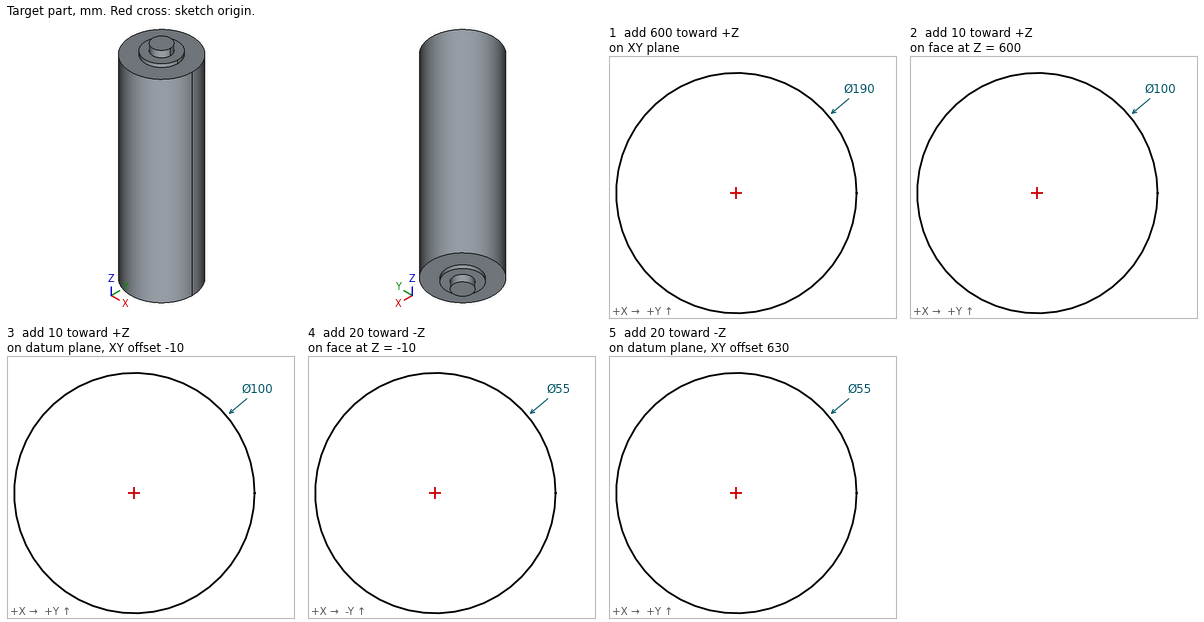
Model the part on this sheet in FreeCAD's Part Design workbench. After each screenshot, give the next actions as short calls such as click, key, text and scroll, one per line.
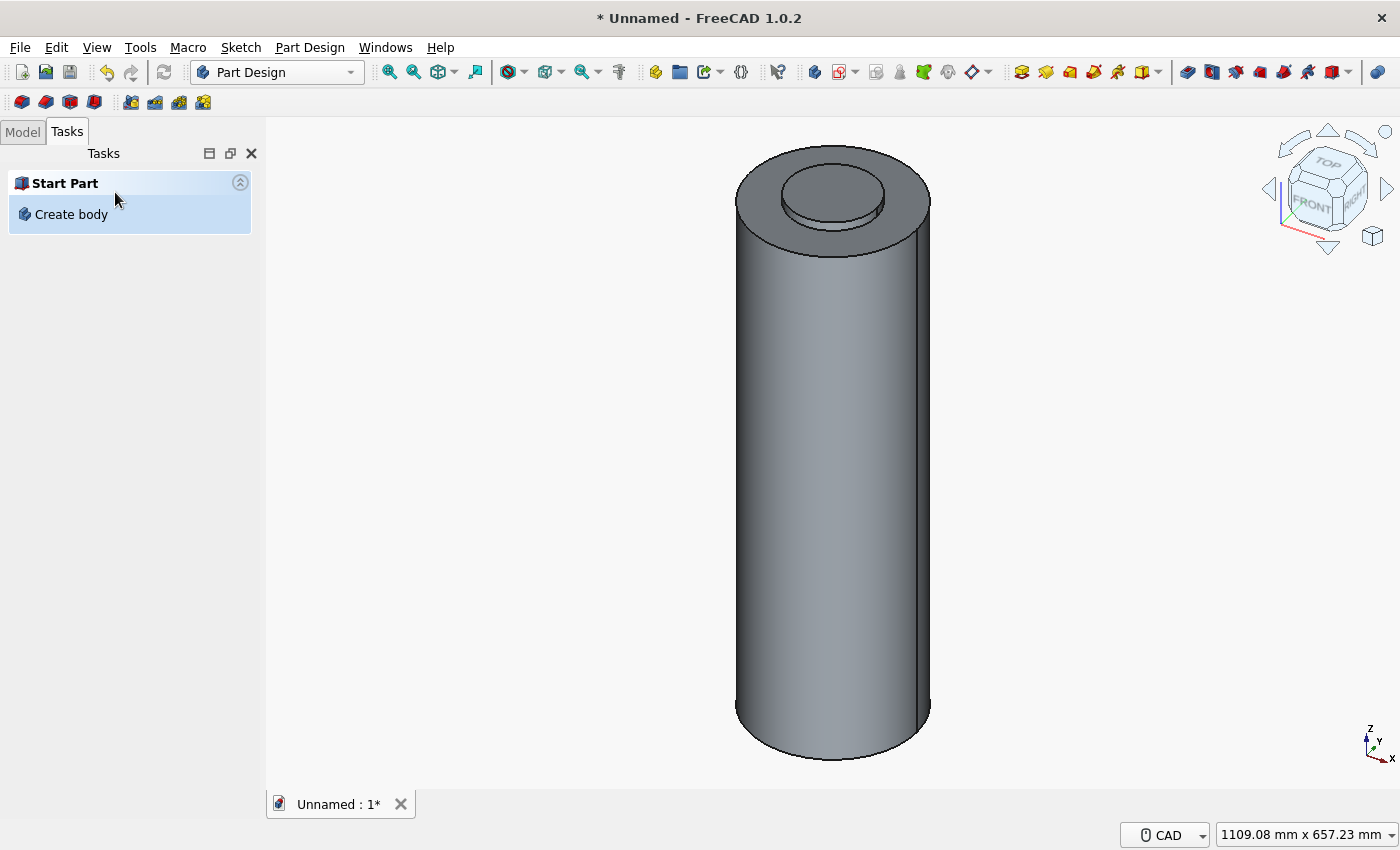
click(390, 72)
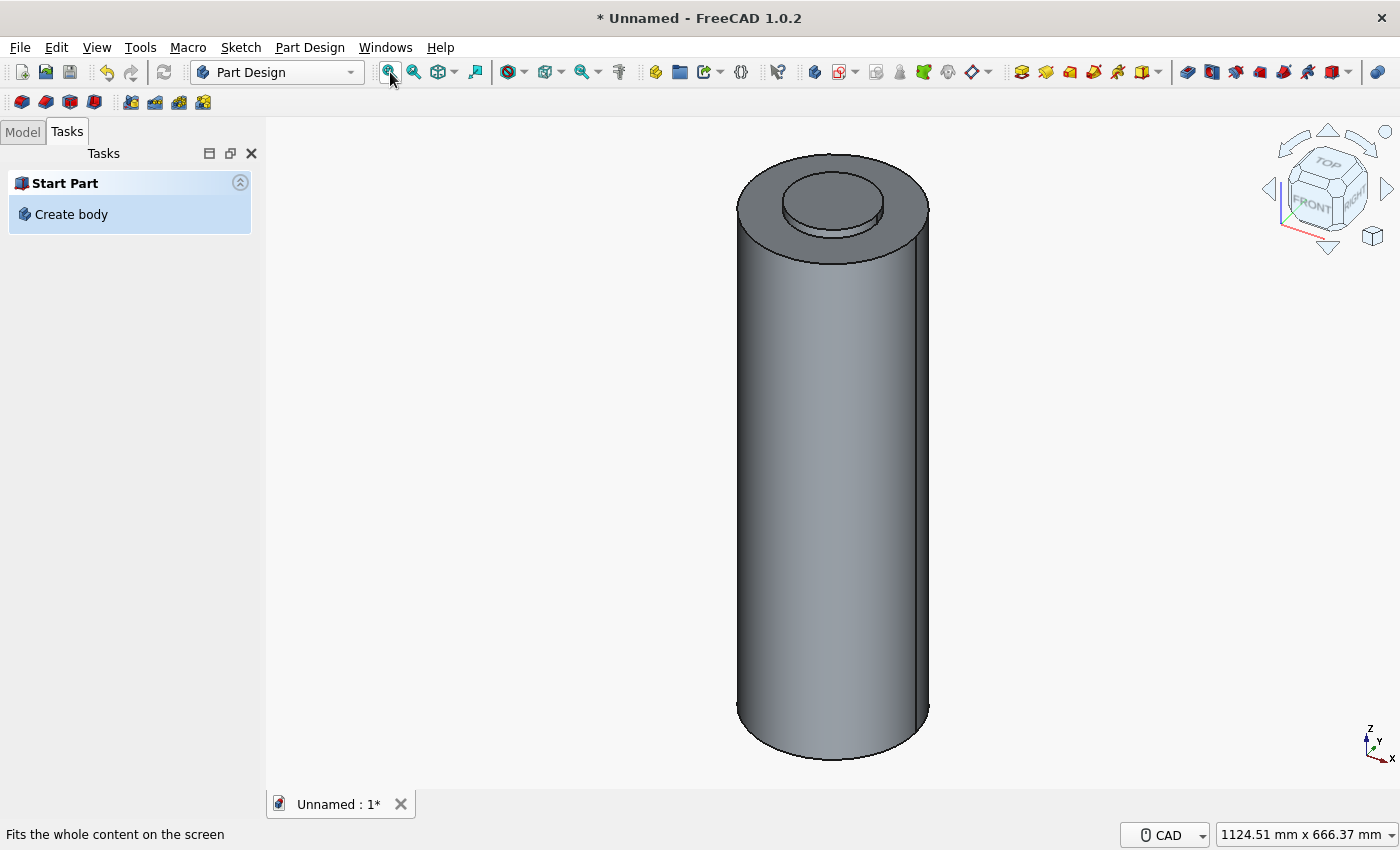
click(23, 131)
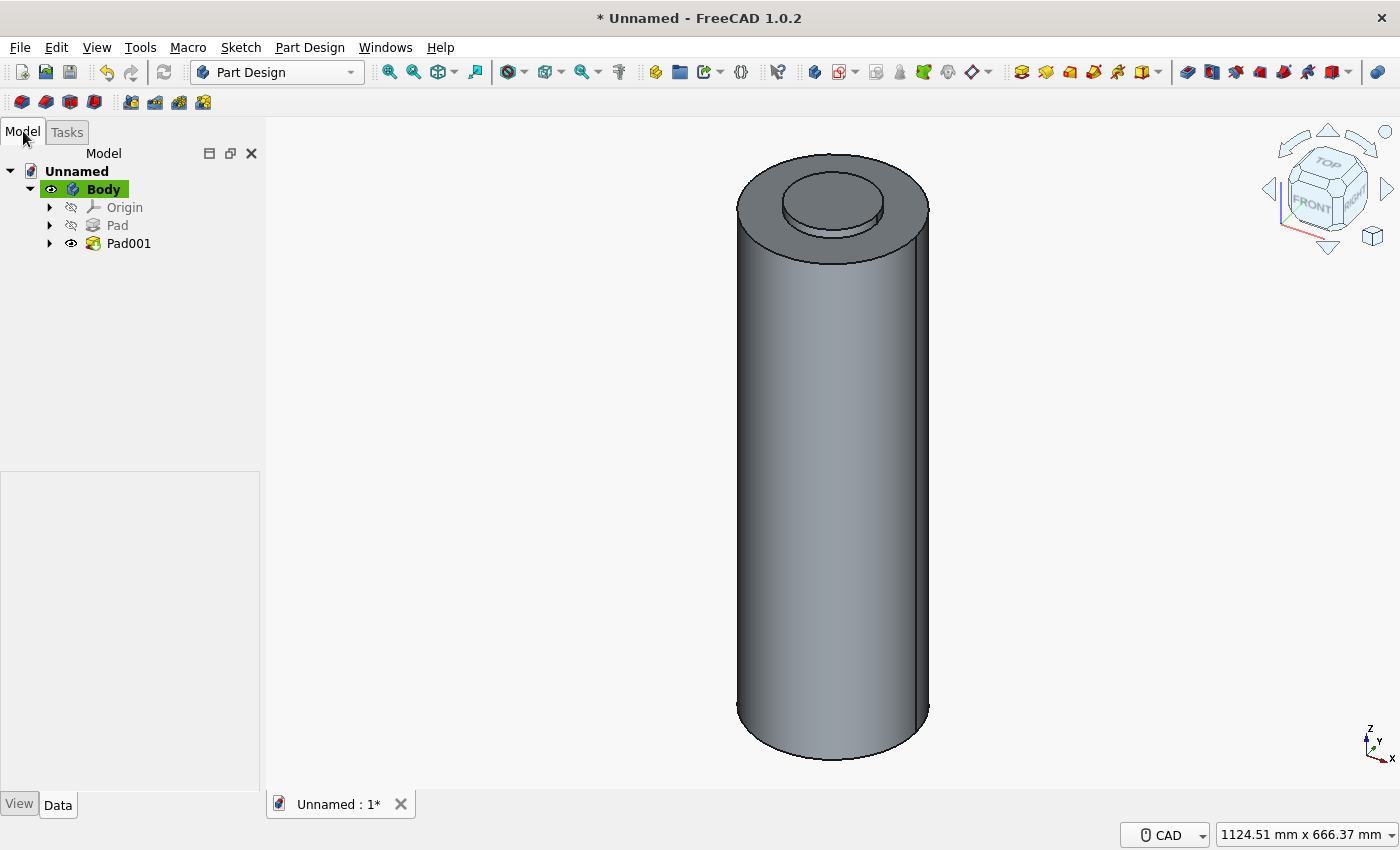
click(50, 207)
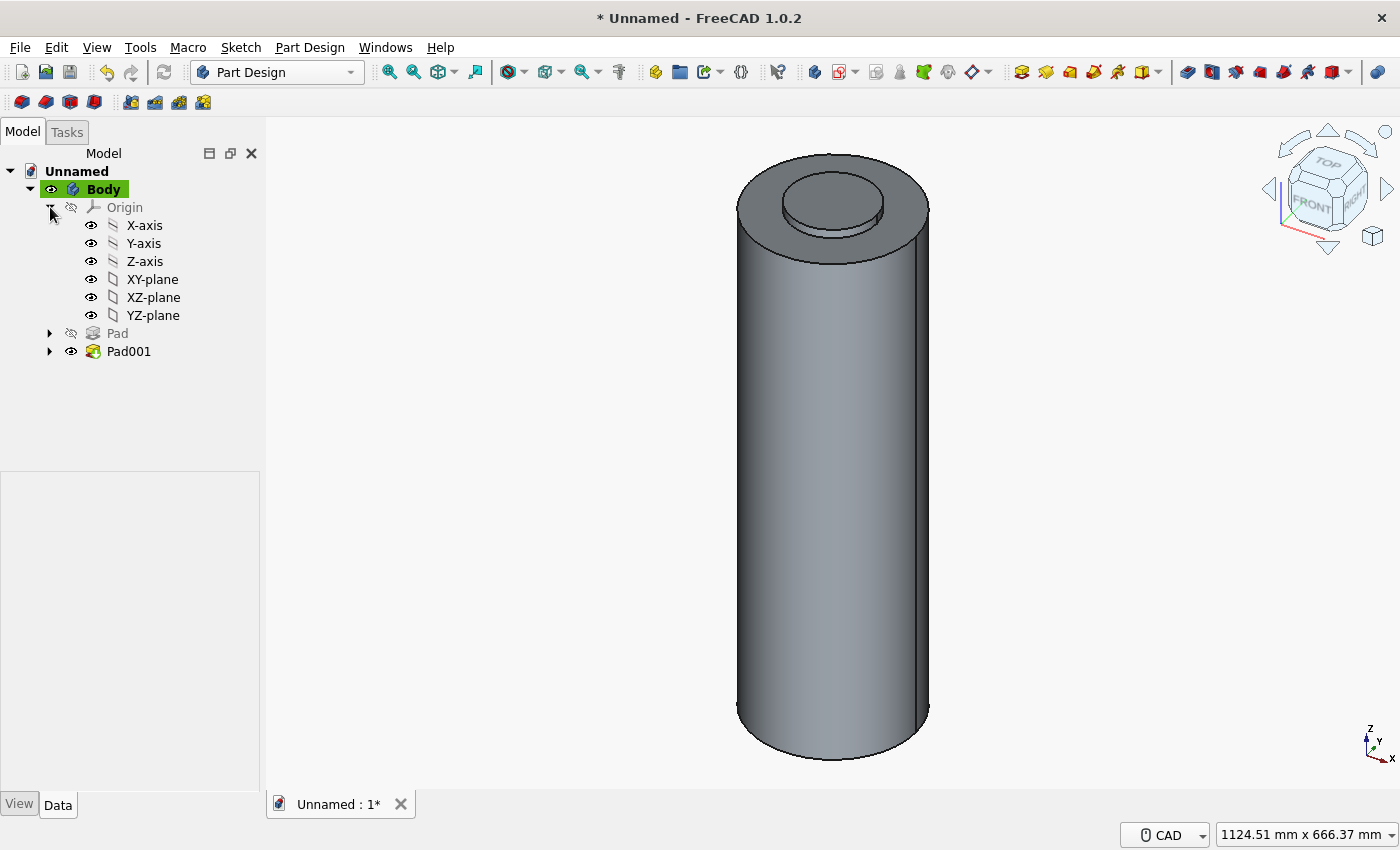
click(136, 279)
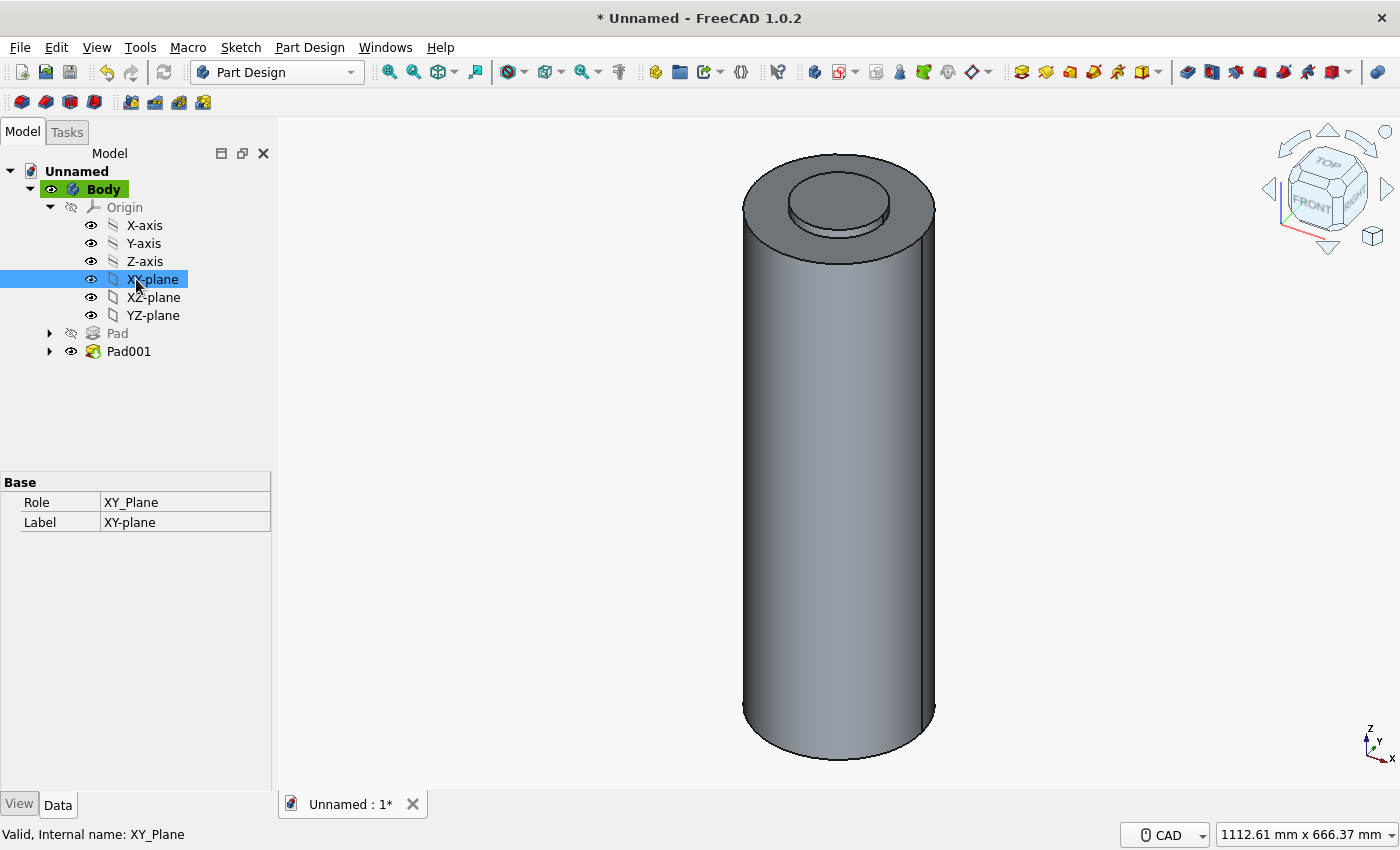
click(972, 72)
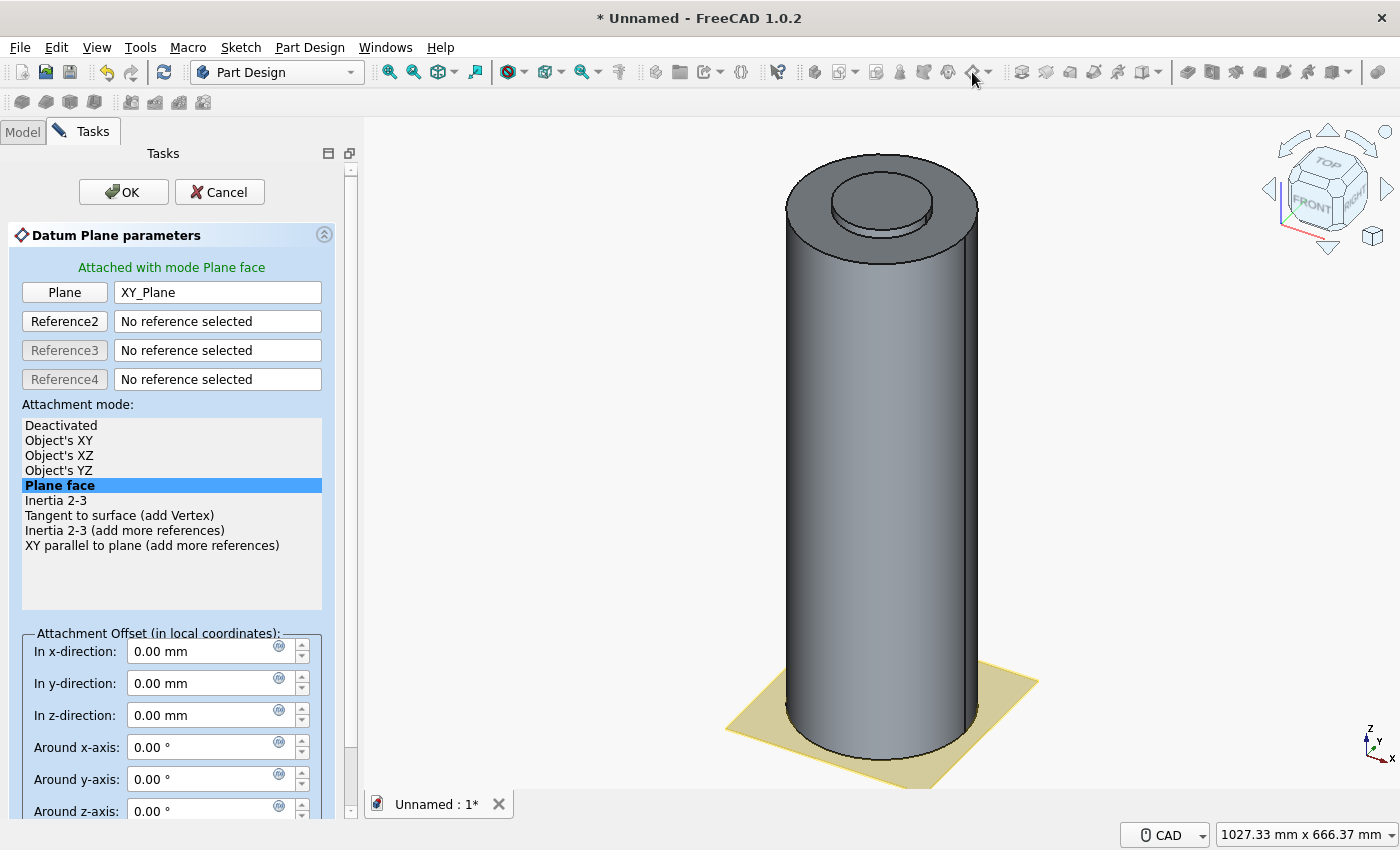
triple_click(210, 715)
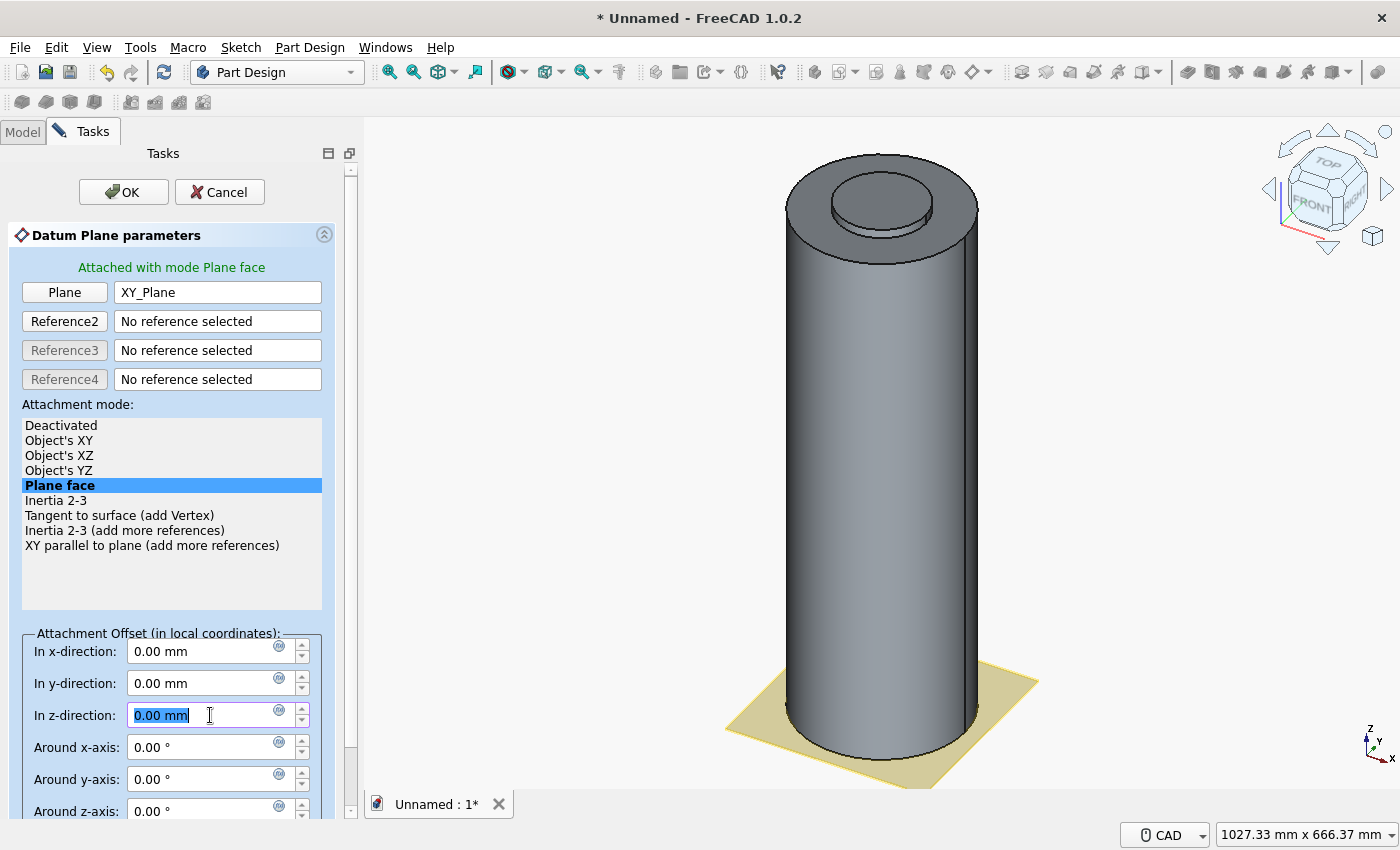
text(-10)
key(Tab)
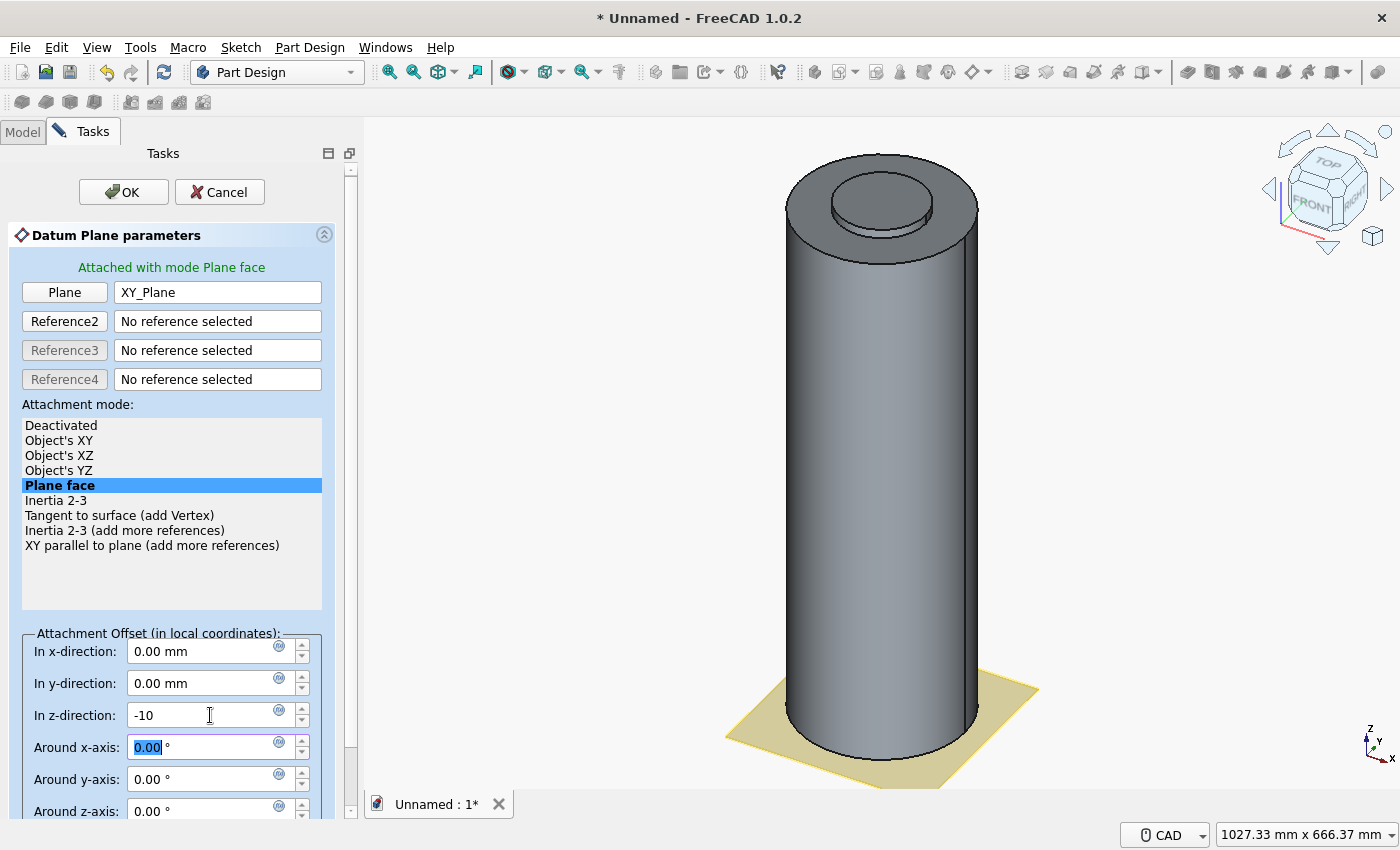
click(124, 192)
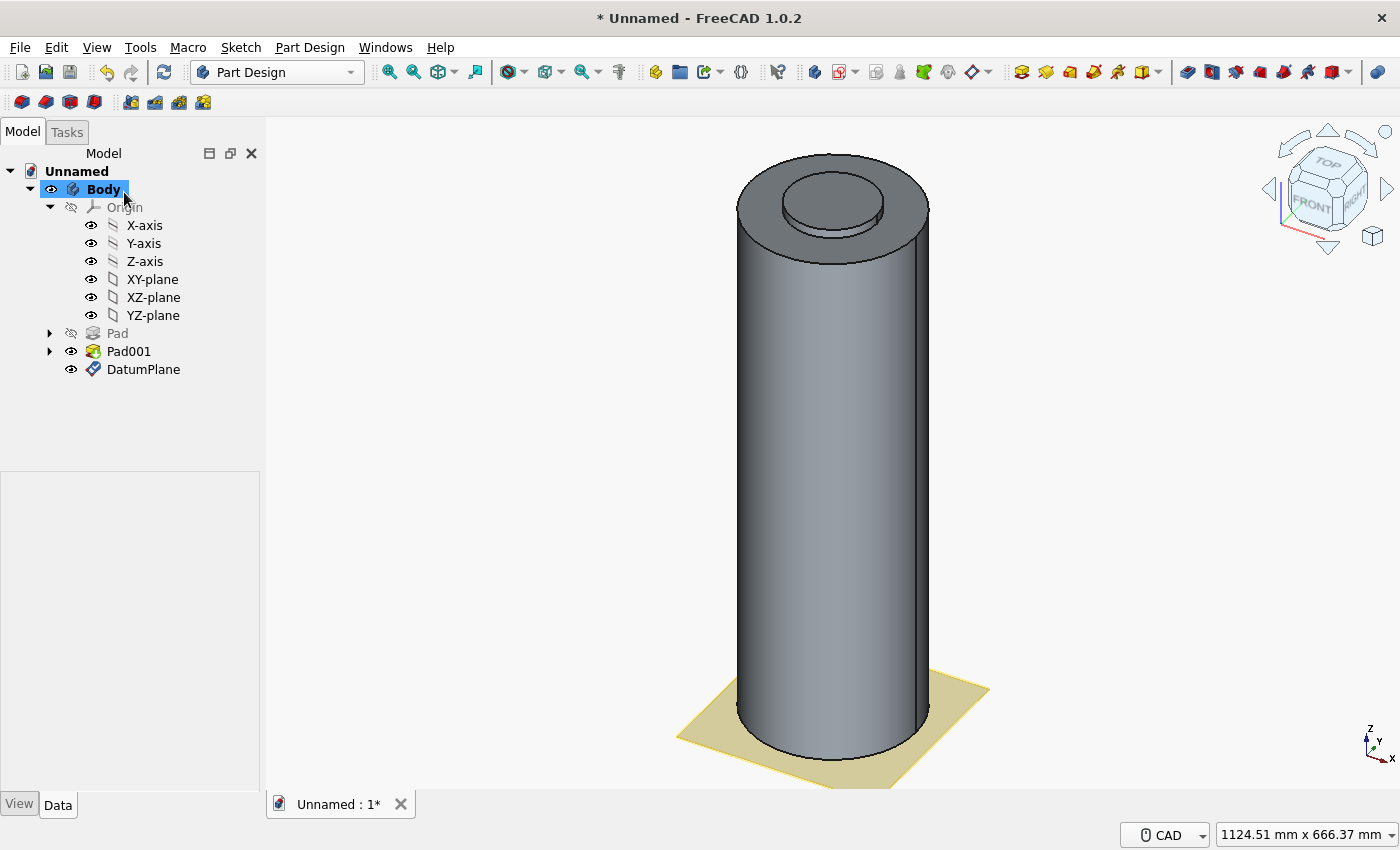
click(116, 369)